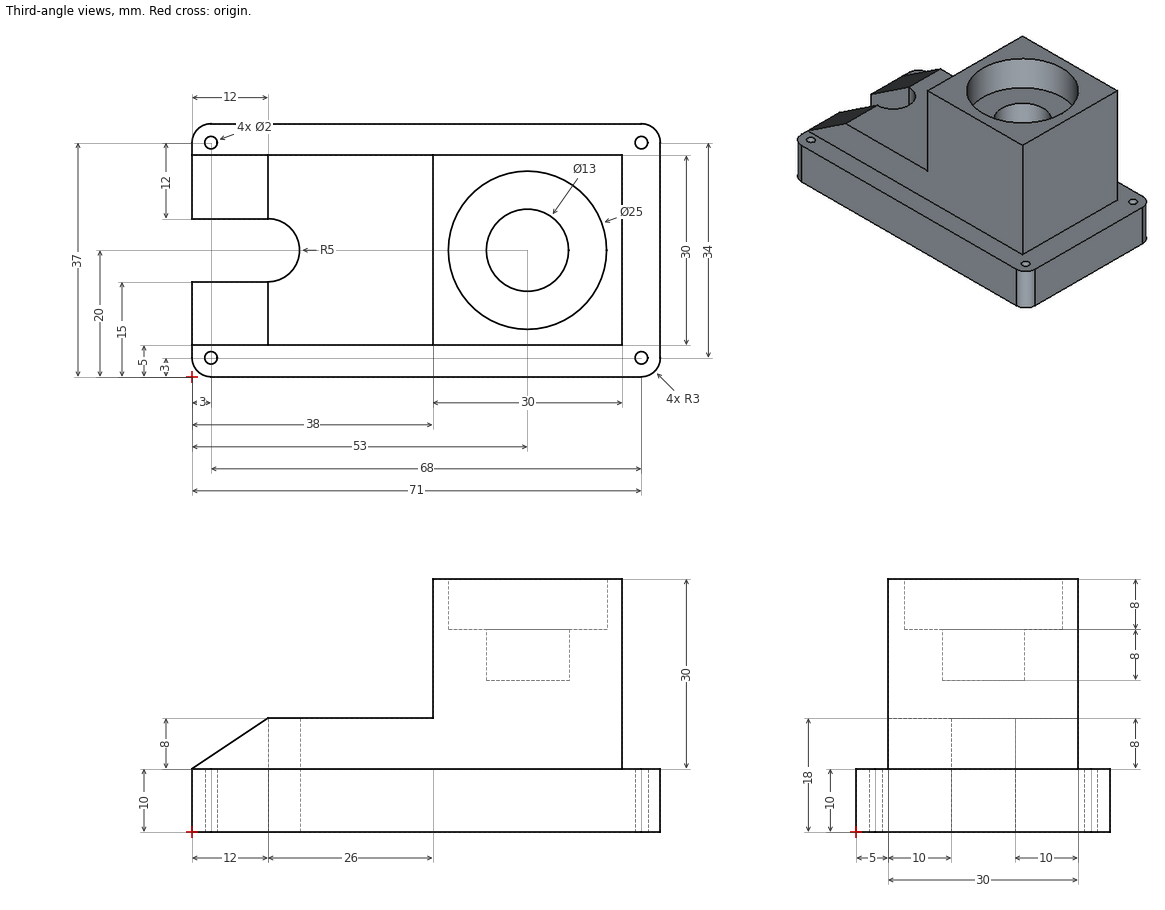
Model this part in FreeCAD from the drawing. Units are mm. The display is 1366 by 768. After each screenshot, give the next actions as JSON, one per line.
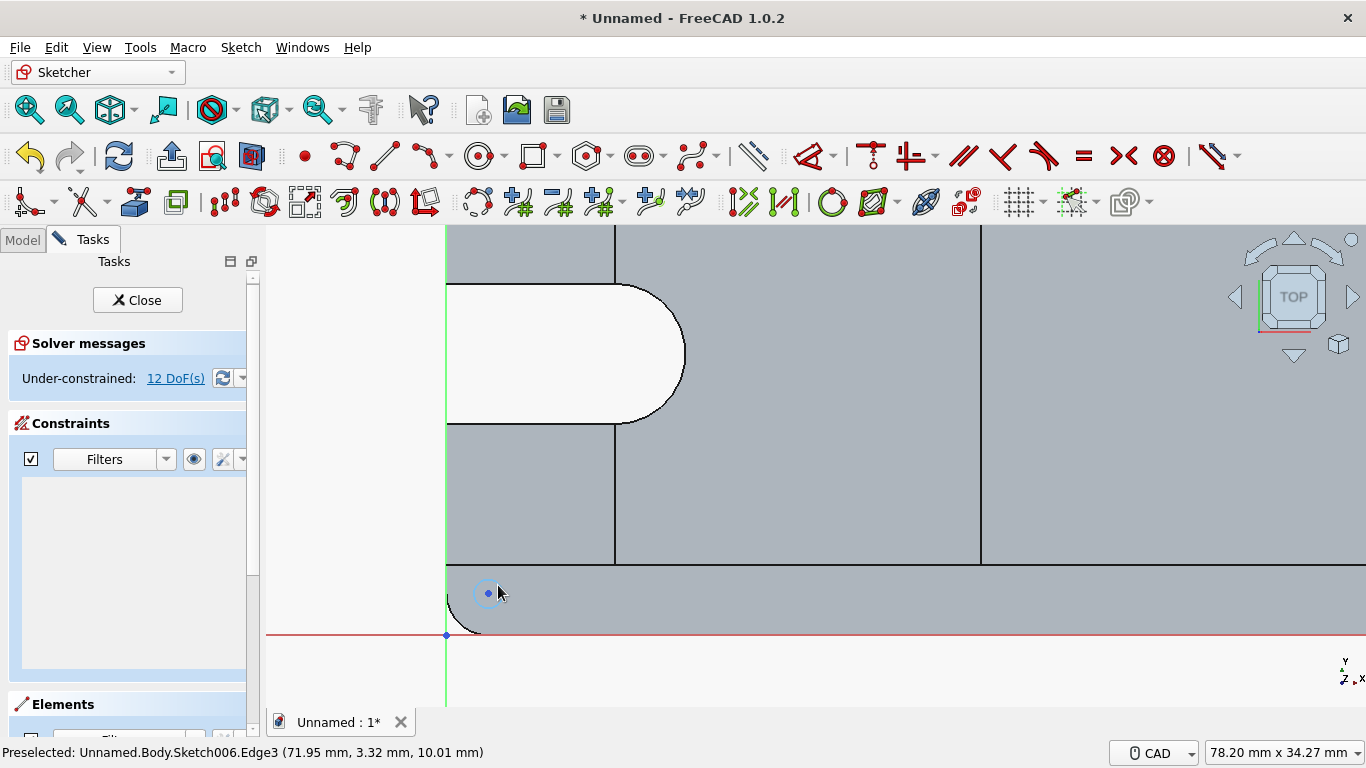
{"action": "left_click", "coordinate": [499, 584]}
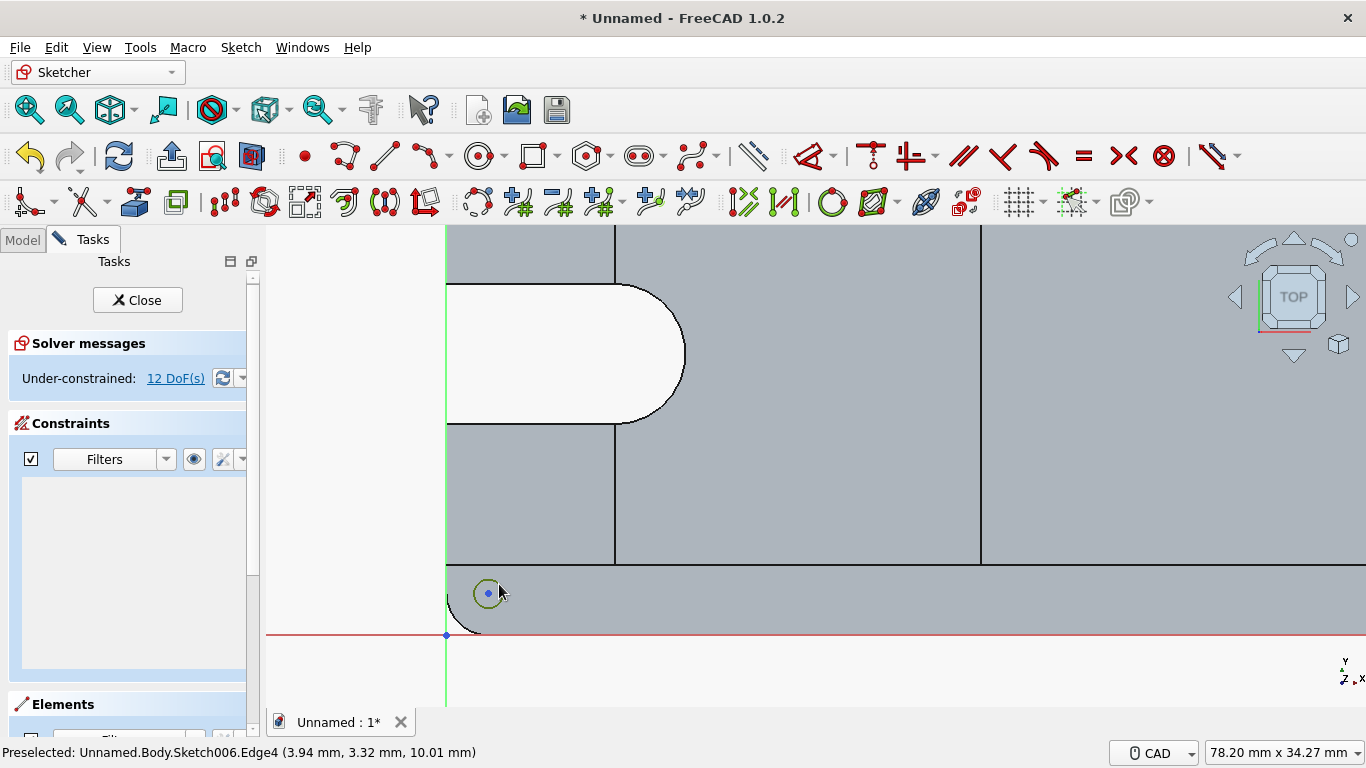
{"action": "left_click", "coordinate": [1084, 156]}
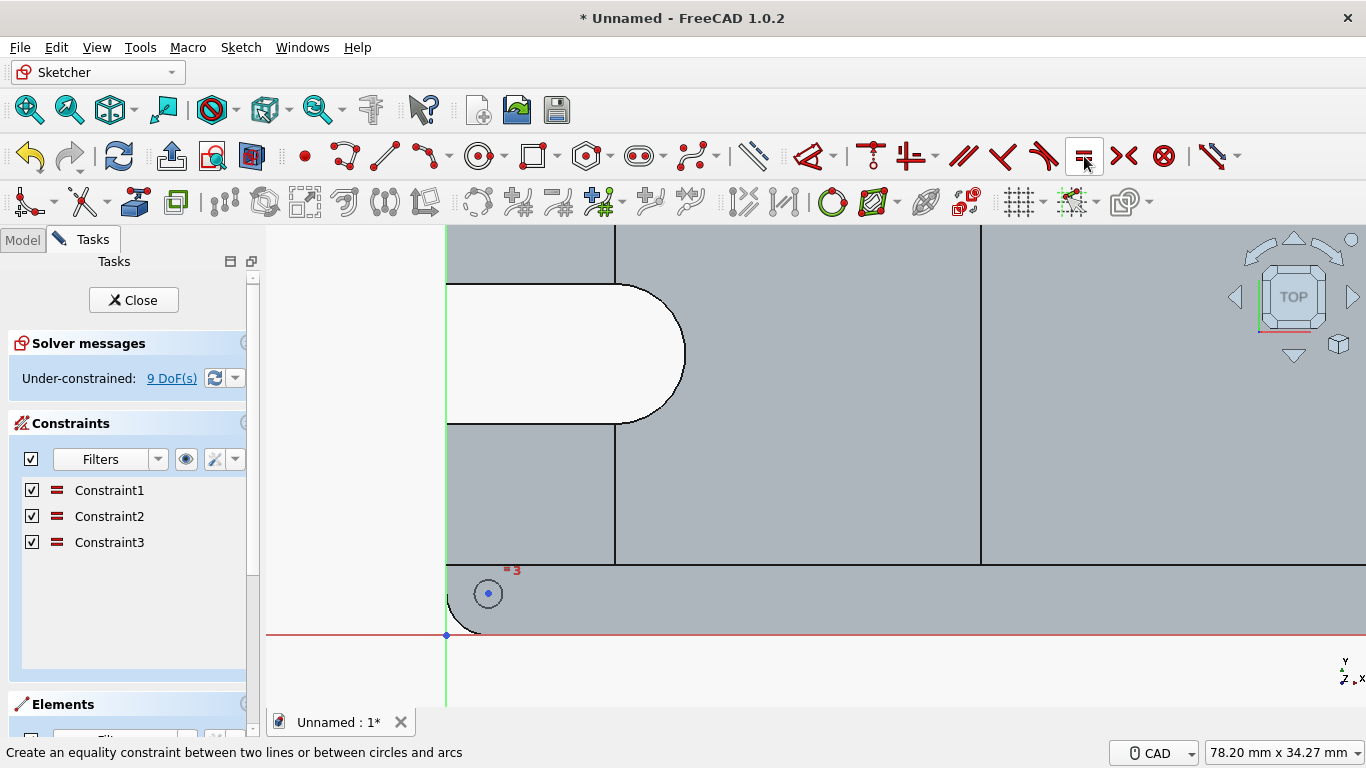
{"action": "scroll", "coordinate": [498, 585], "scroll_direction": "down", "scroll_amount": 3}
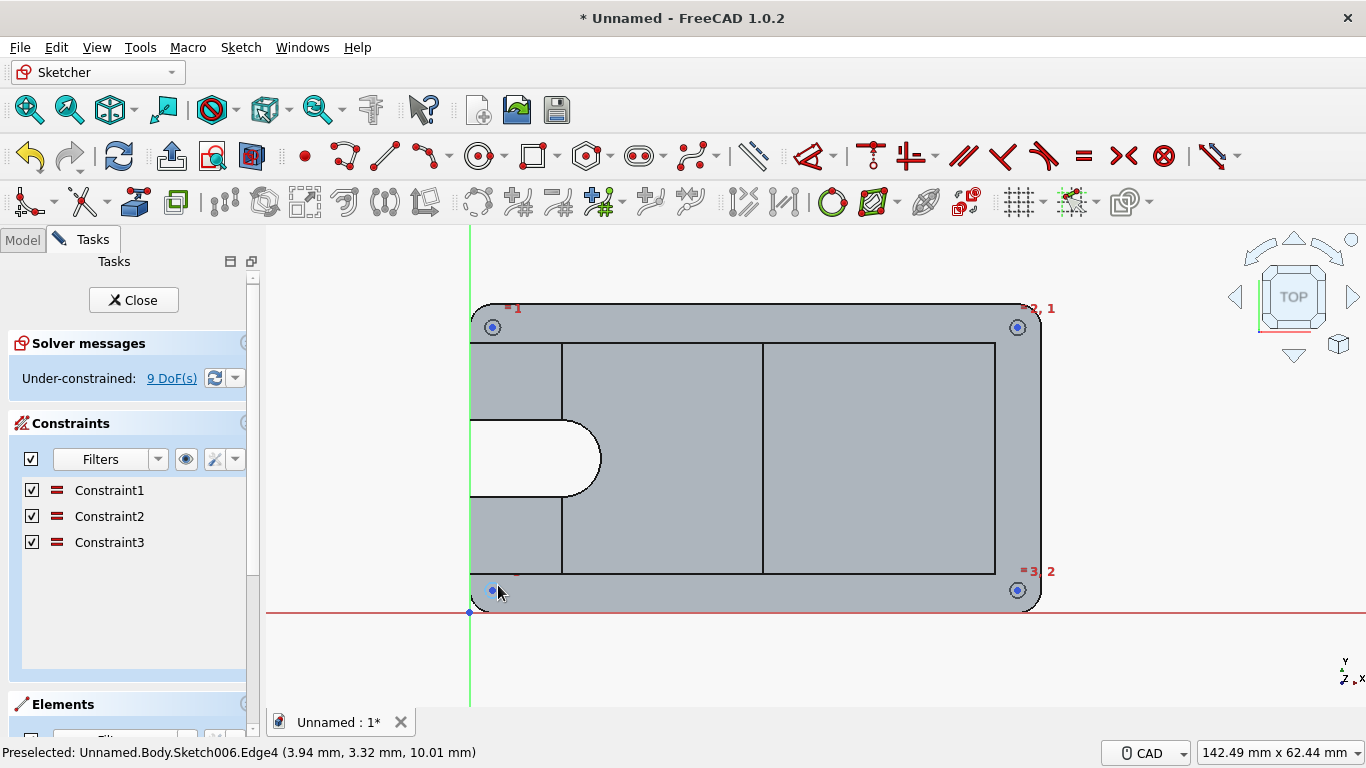
{"action": "left_click", "coordinate": [493, 328]}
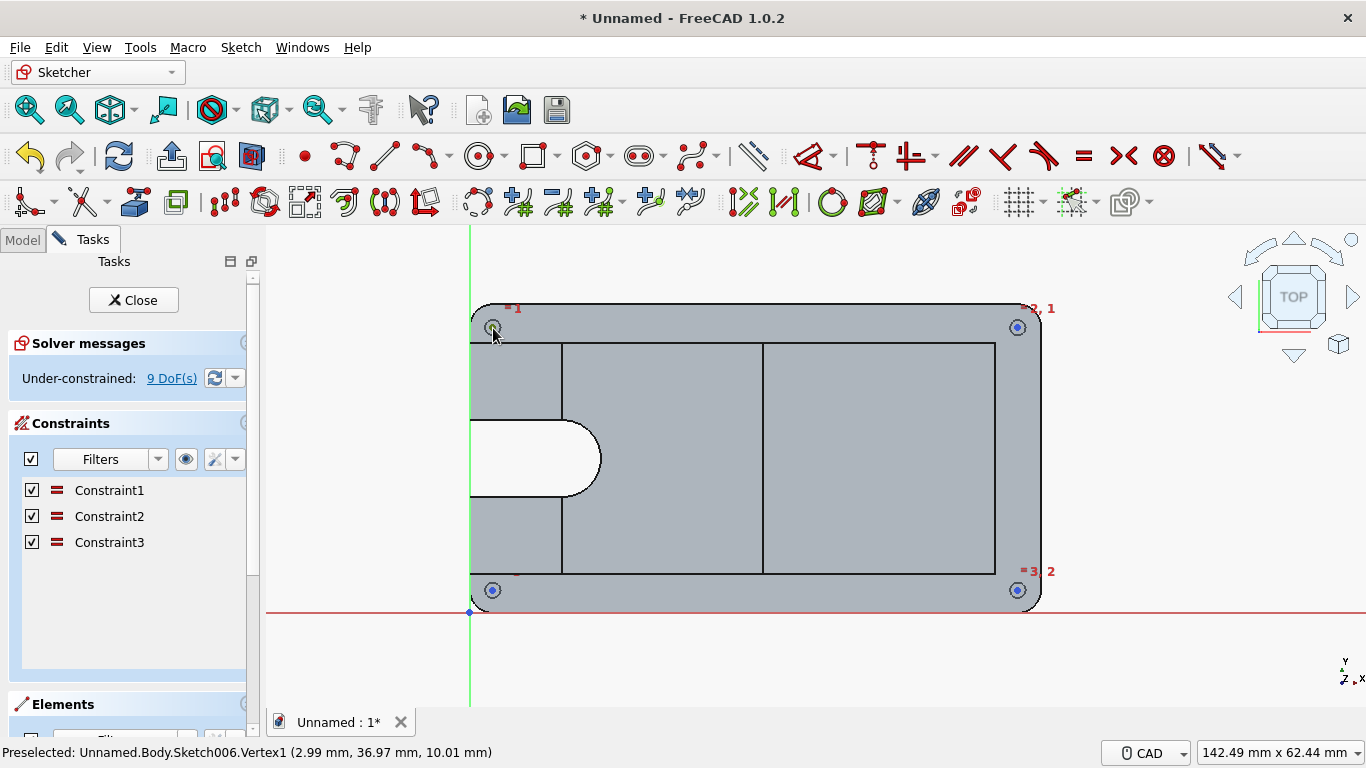
{"action": "left_click", "coordinate": [1018, 328]}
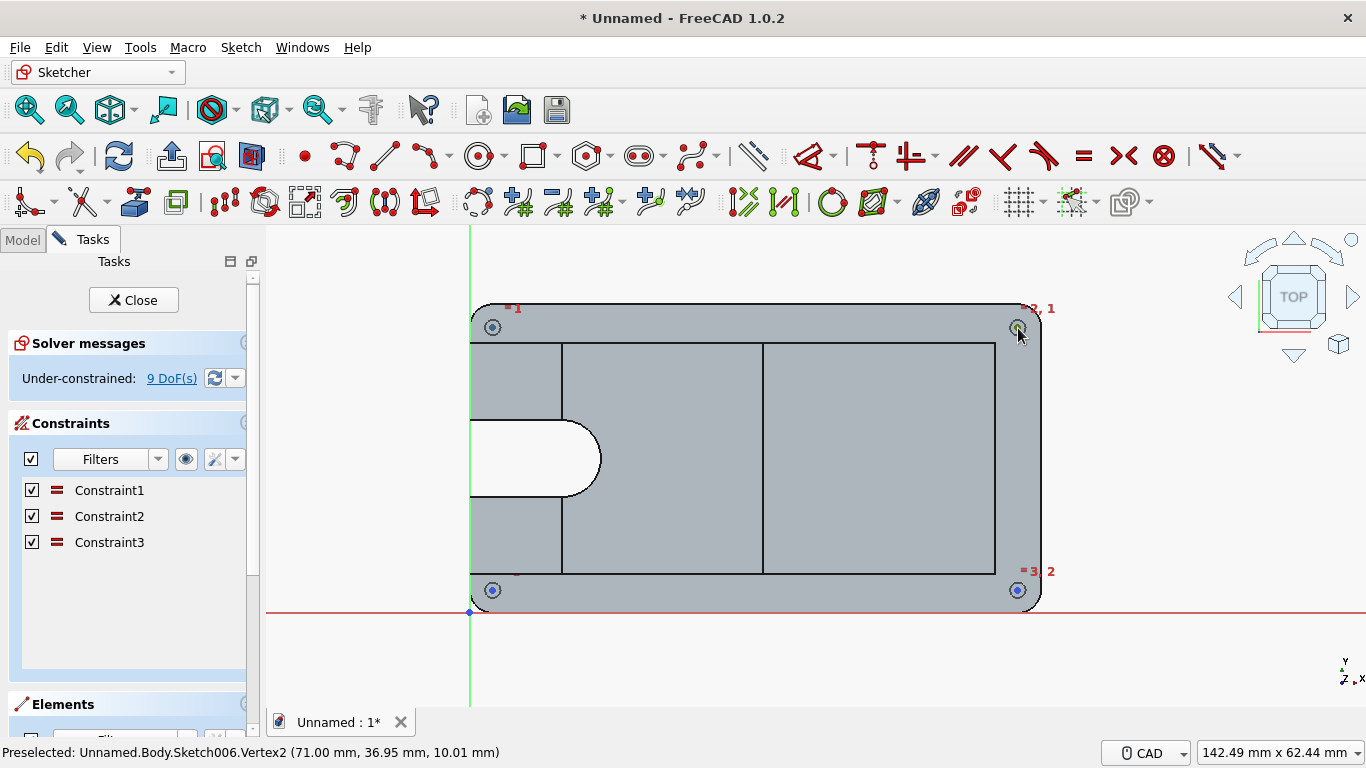
{"action": "key", "text": "h"}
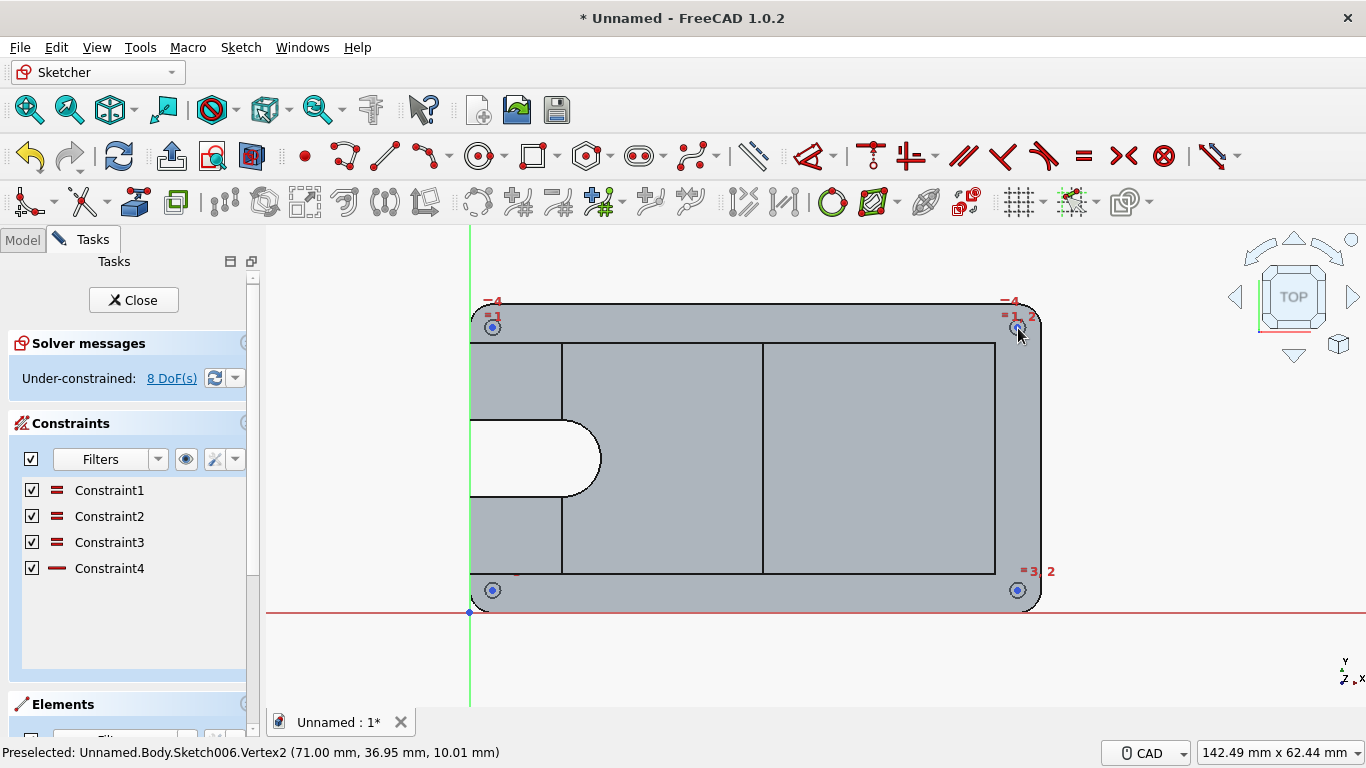
{"action": "left_click", "coordinate": [1018, 328]}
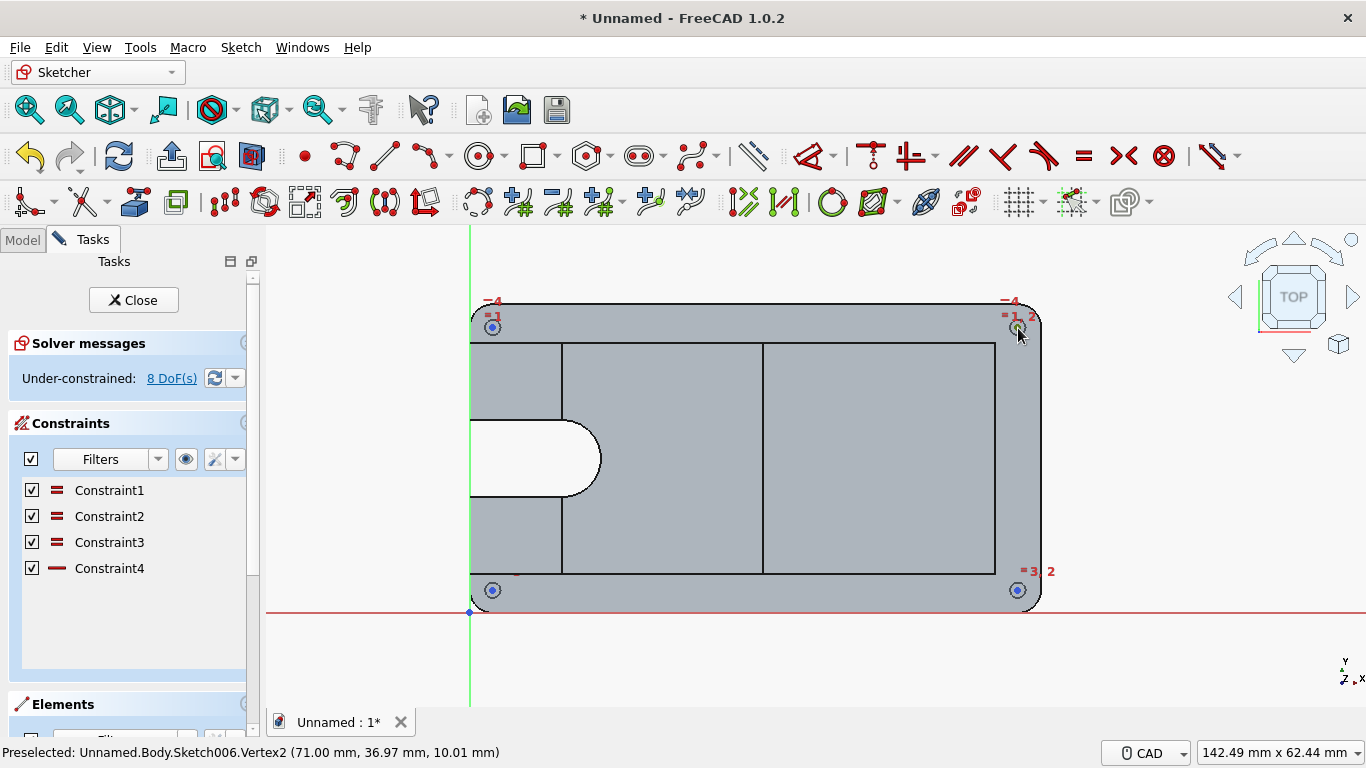
{"action": "left_click", "coordinate": [1018, 590]}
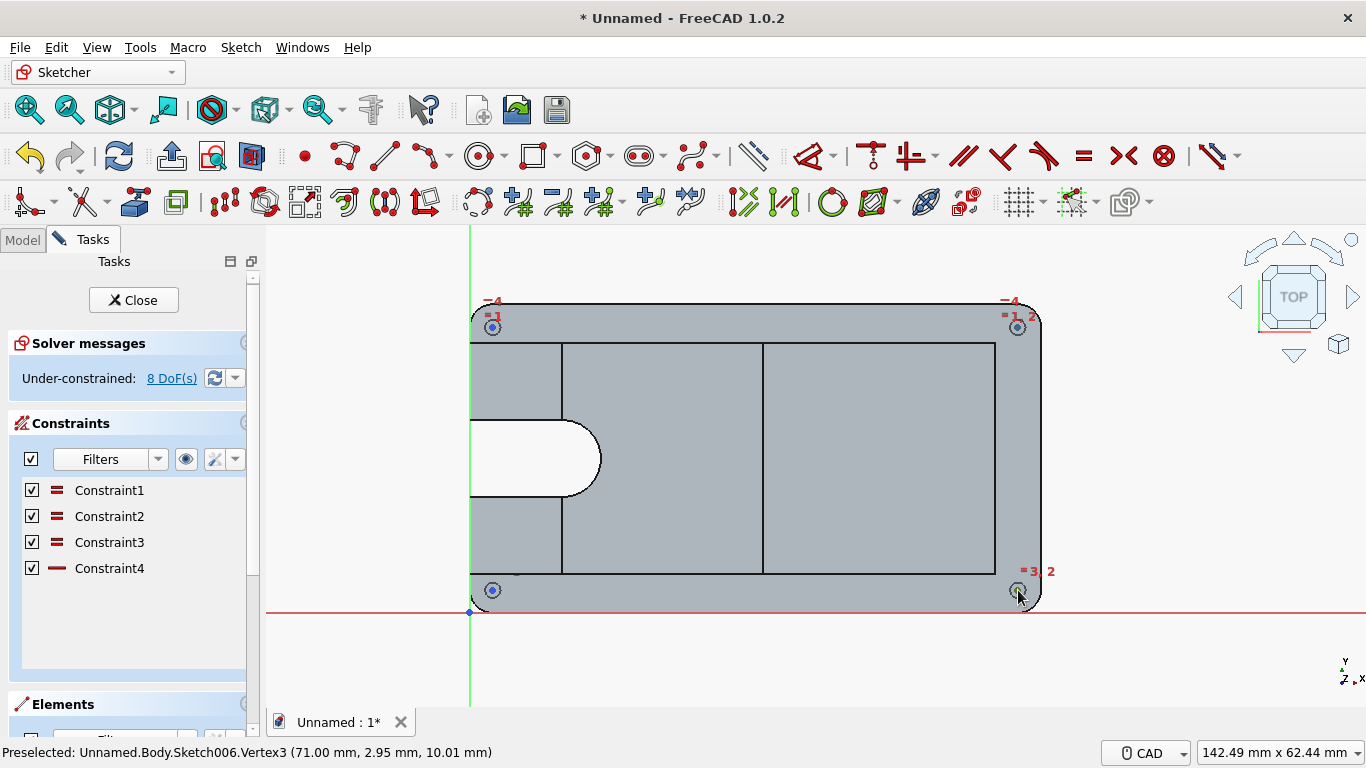
{"action": "left_click", "coordinate": [938, 156]}